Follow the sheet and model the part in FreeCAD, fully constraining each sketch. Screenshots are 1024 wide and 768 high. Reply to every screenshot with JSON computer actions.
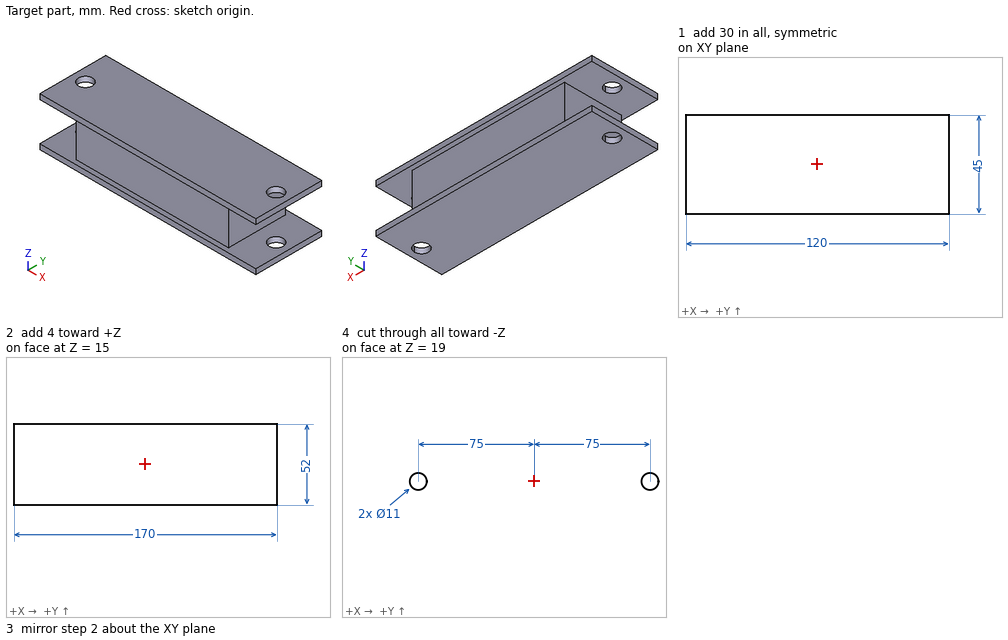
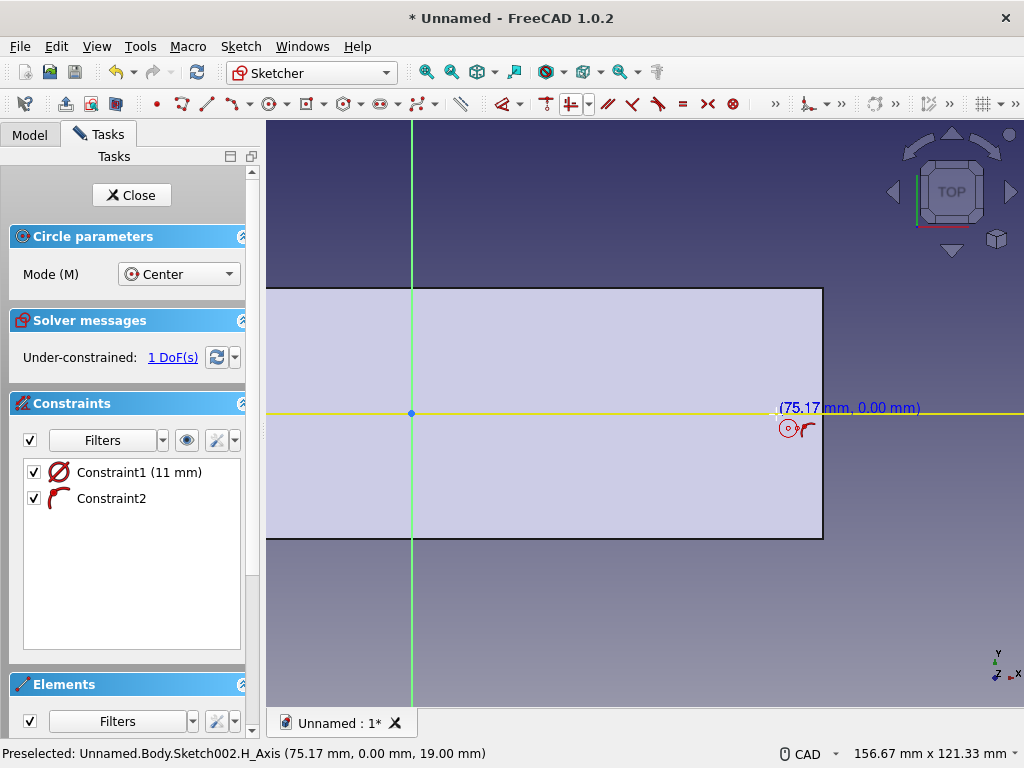
{"action": "left_click", "coordinate": [775, 414]}
{"action": "mouse_move", "coordinate": [793, 395]}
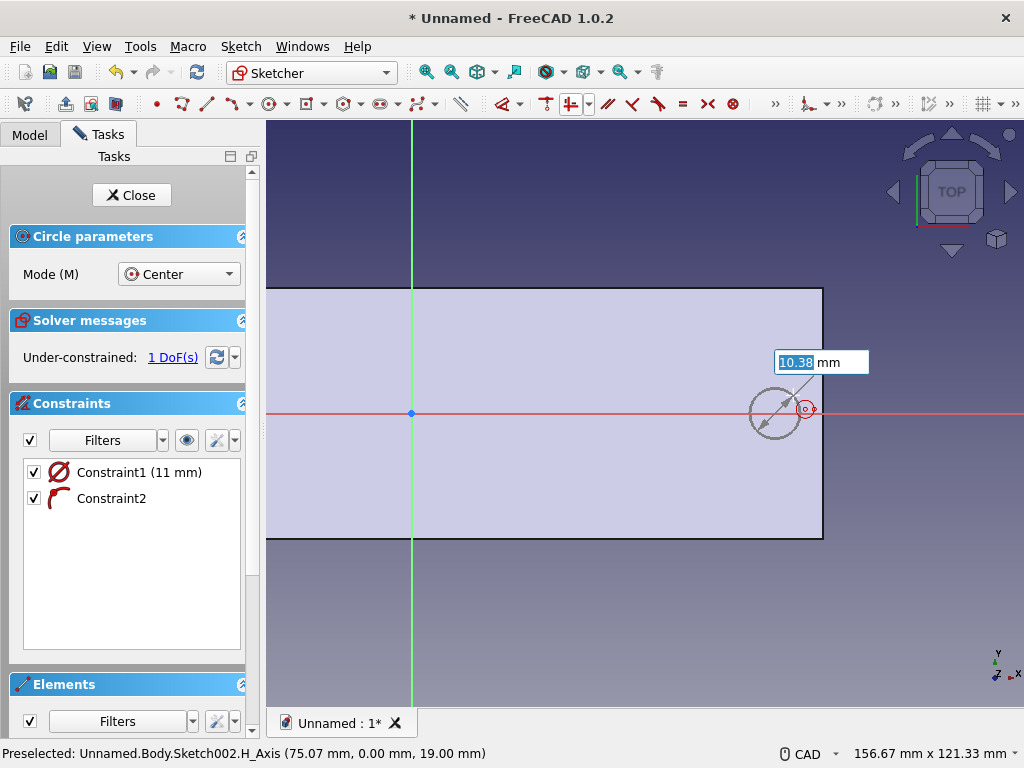
{"action": "type", "text": "11"}
{"action": "key", "text": "Return"}
{"action": "key", "text": "Escape"}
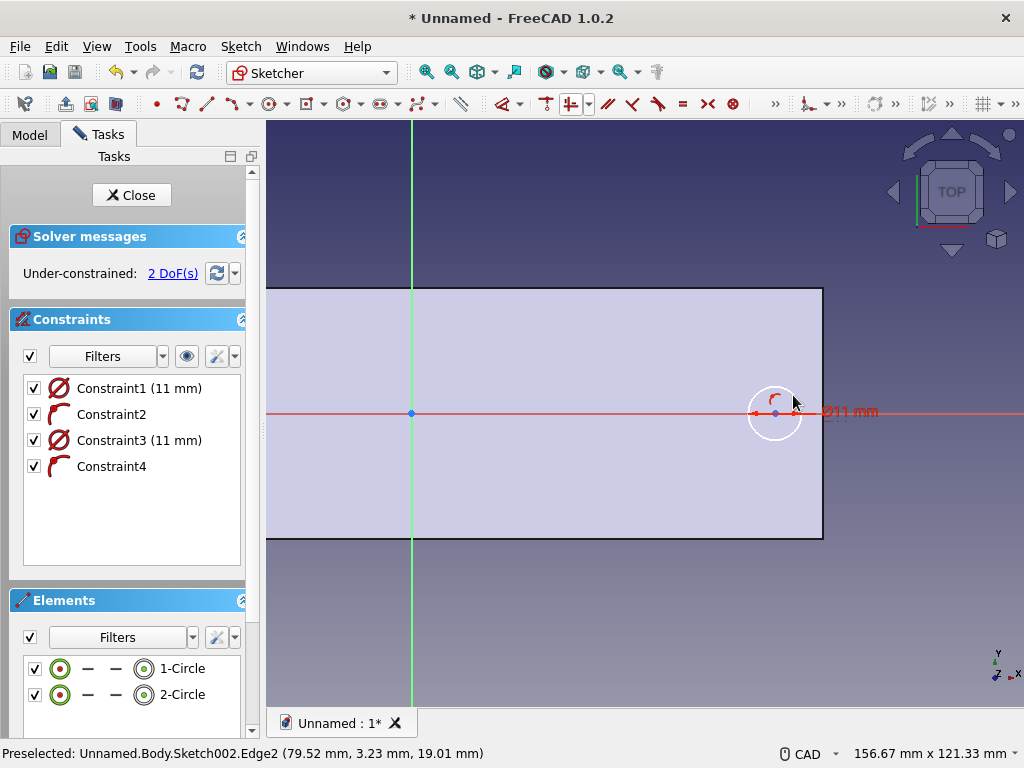
{"action": "left_click", "coordinate": [502, 104]}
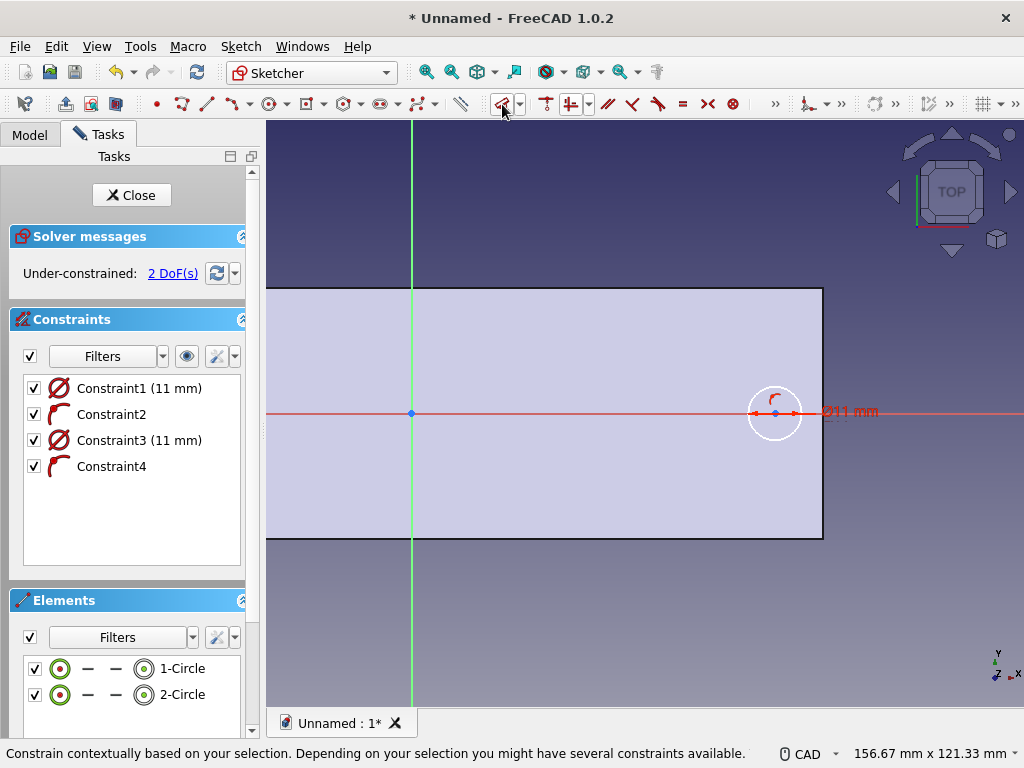
{"action": "scroll", "coordinate": [777, 413], "scroll_direction": "down", "scroll_amount": 3}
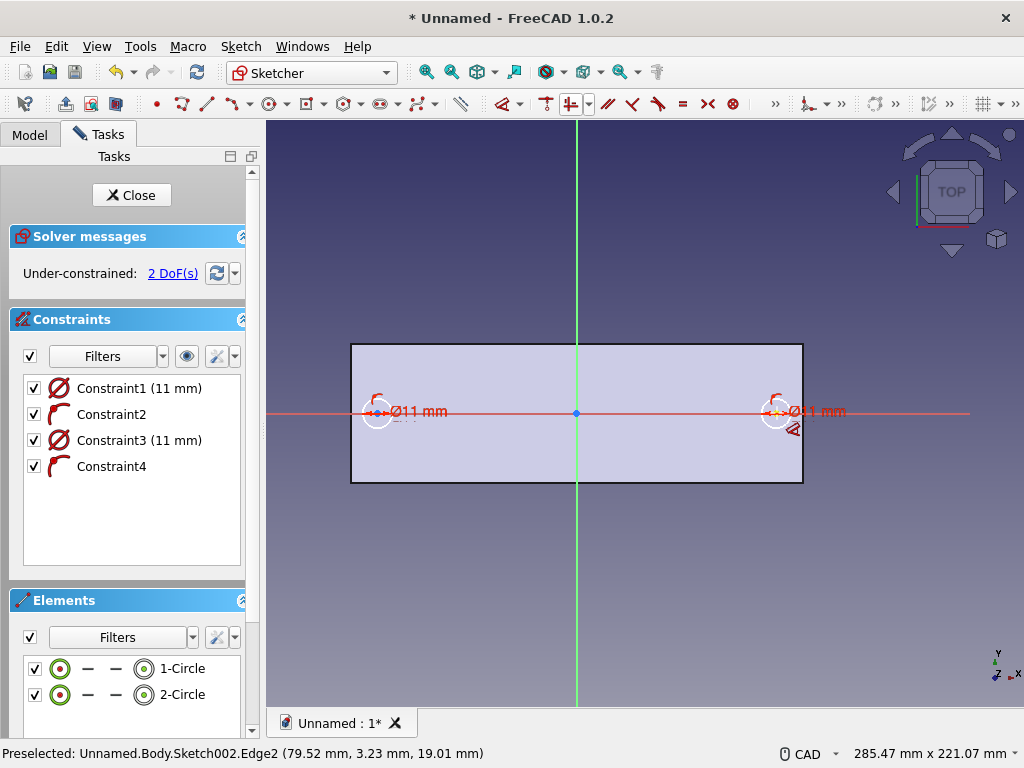
{"action": "left_click", "coordinate": [378, 414]}
{"action": "left_click", "coordinate": [477, 448]}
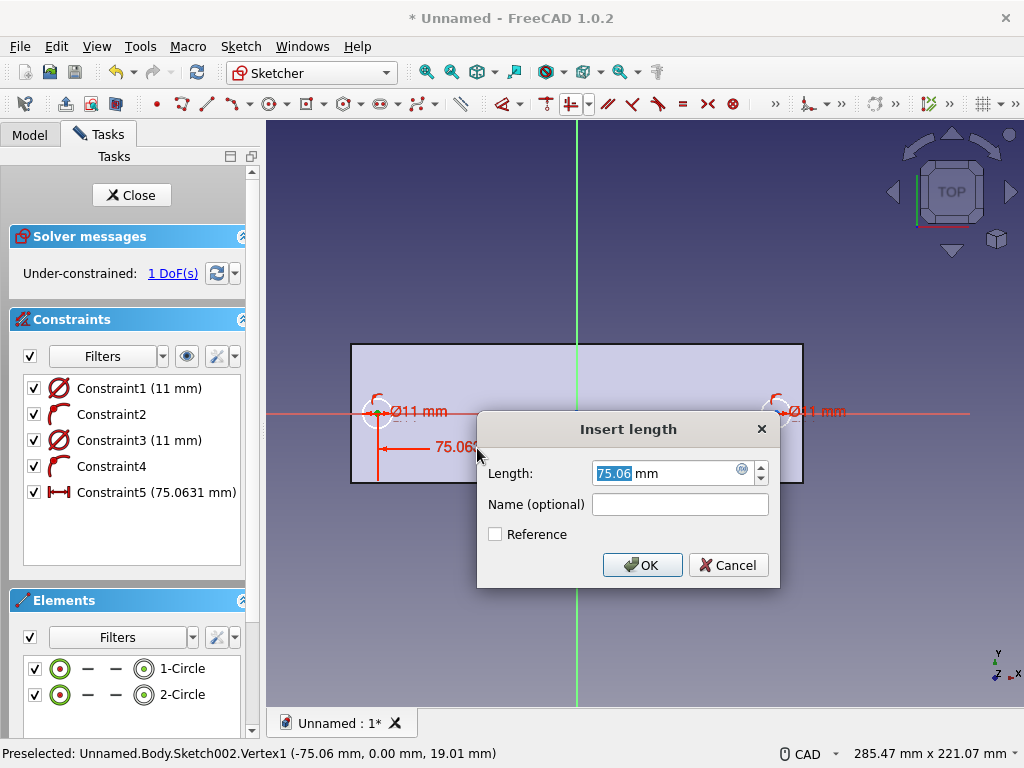
{"action": "type", "text": "75"}
{"action": "key", "text": "Return"}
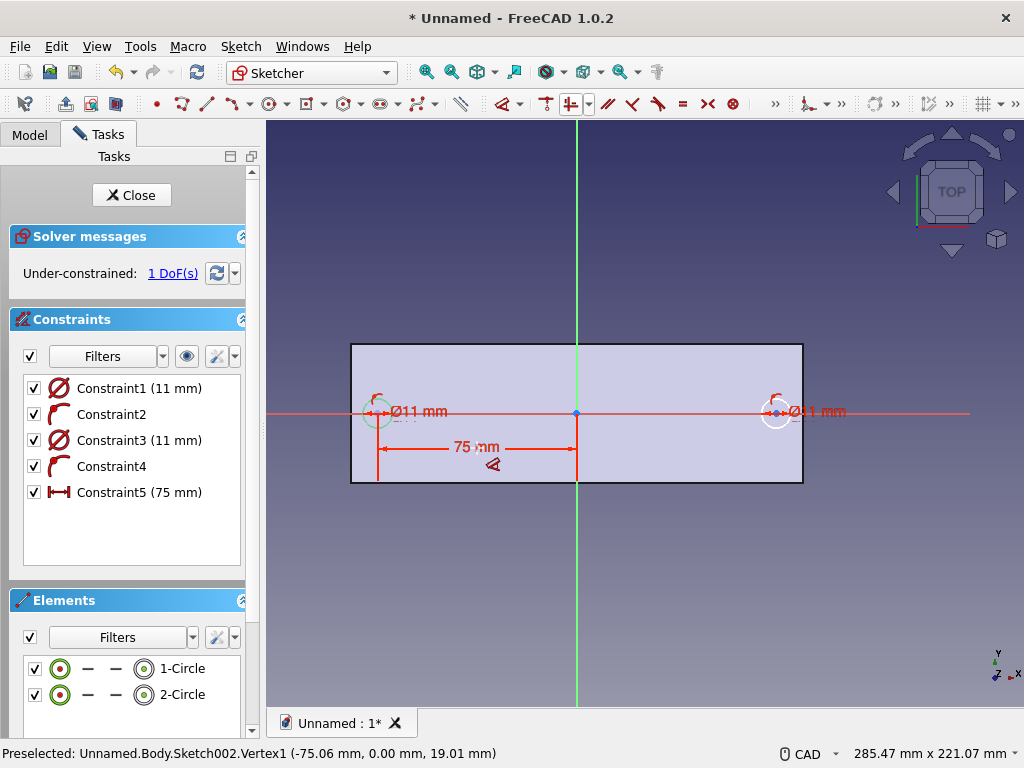
{"action": "left_click", "coordinate": [776, 414]}
{"action": "left_click", "coordinate": [677, 448]}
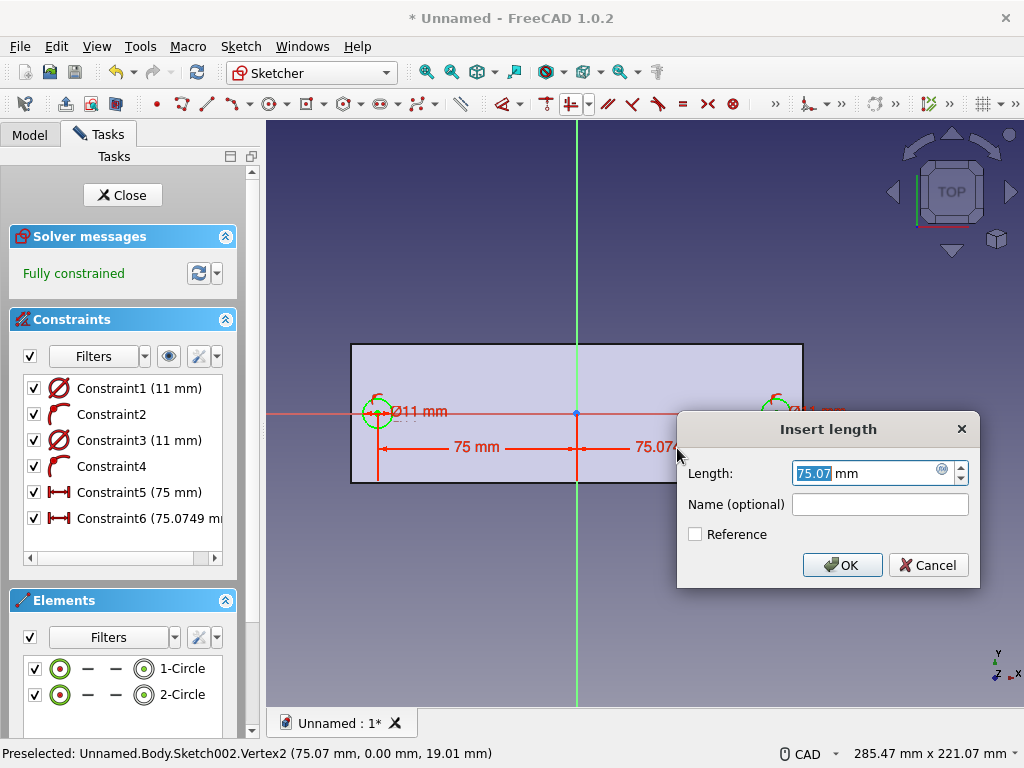
{"action": "type", "text": "75"}
{"action": "key", "text": "Return"}
{"action": "key", "text": "Escape"}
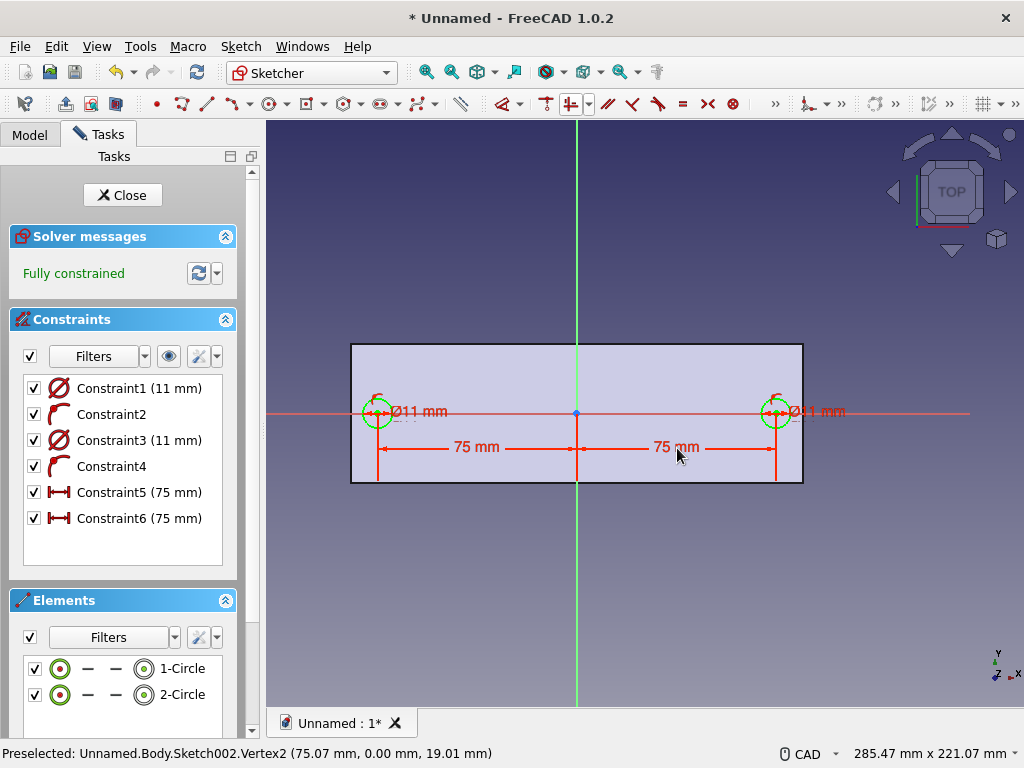
{"action": "left_click", "coordinate": [123, 195]}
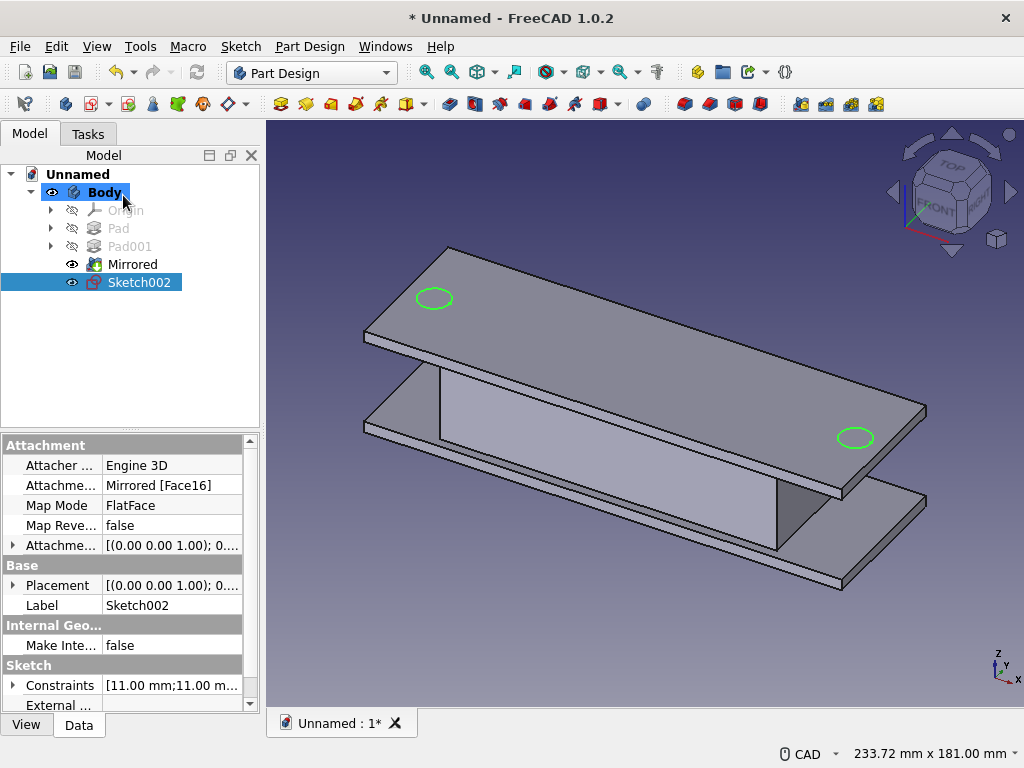
{"action": "left_click", "coordinate": [450, 104]}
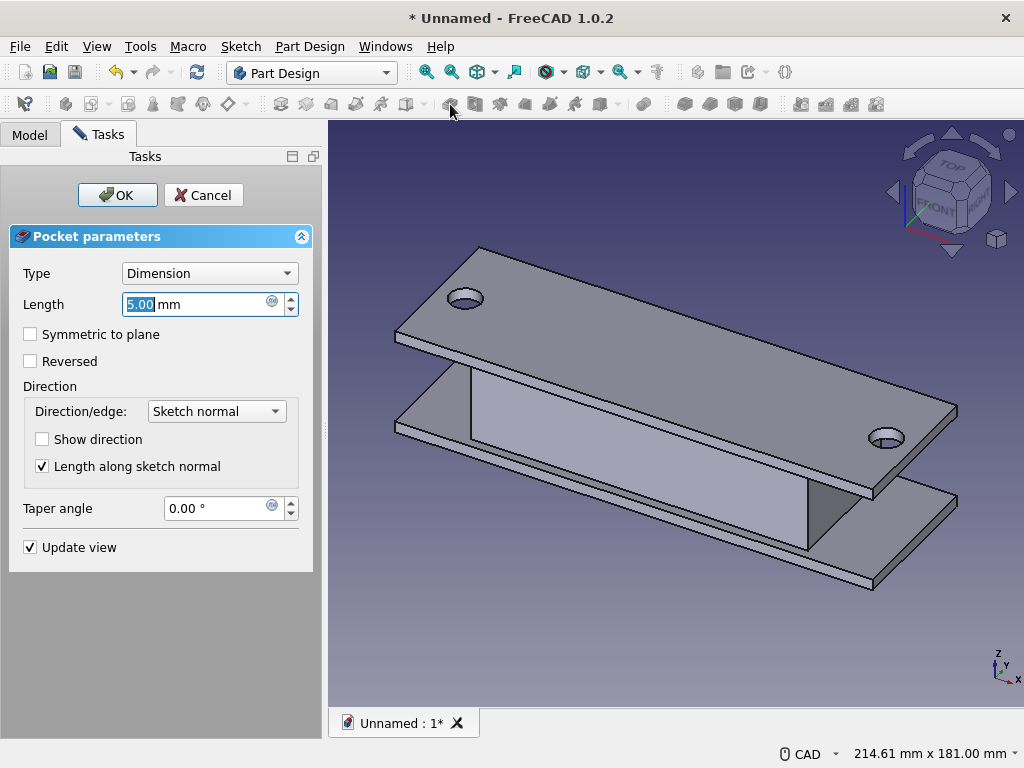
{"action": "left_click", "coordinate": [210, 274]}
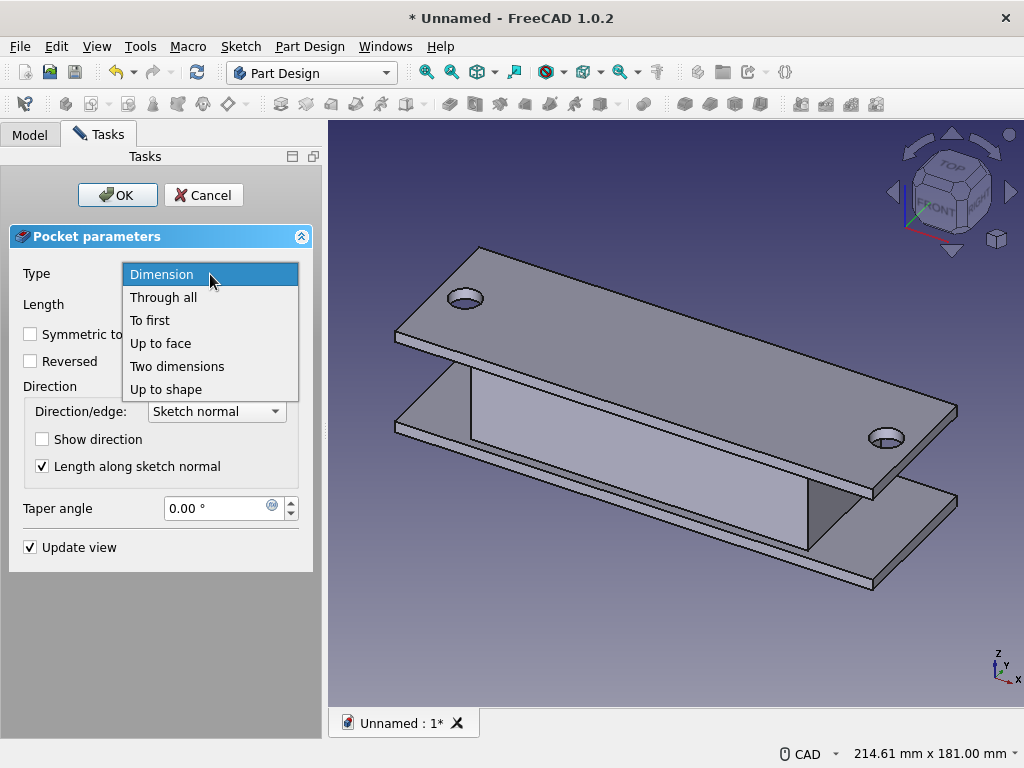
{"action": "left_click", "coordinate": [208, 298]}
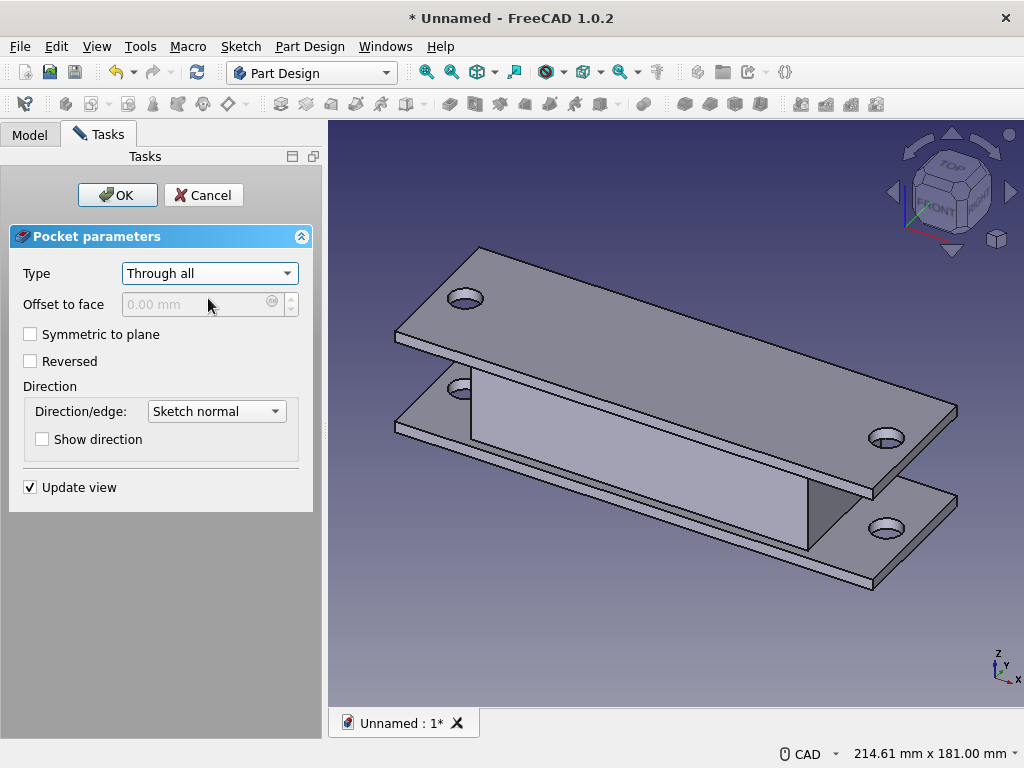
{"action": "left_click", "coordinate": [118, 195]}